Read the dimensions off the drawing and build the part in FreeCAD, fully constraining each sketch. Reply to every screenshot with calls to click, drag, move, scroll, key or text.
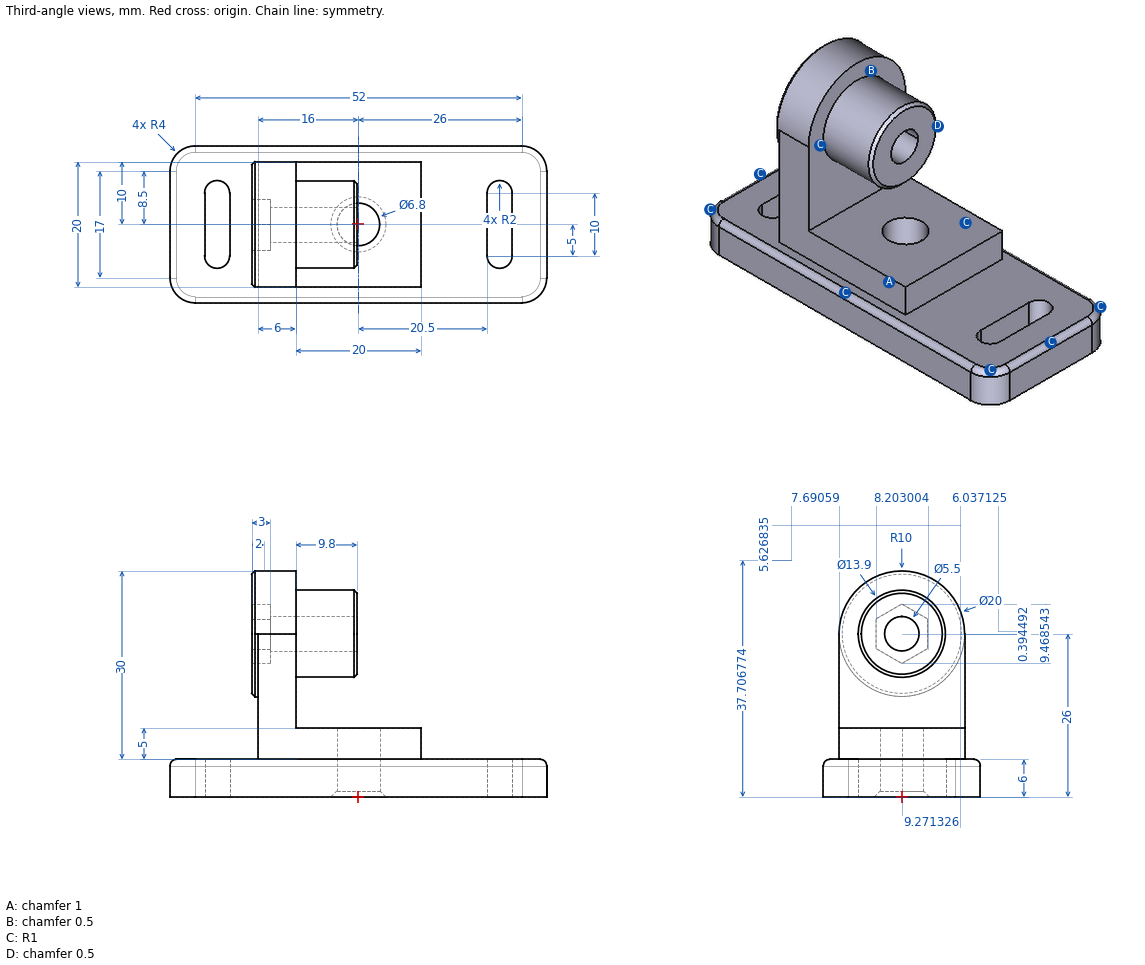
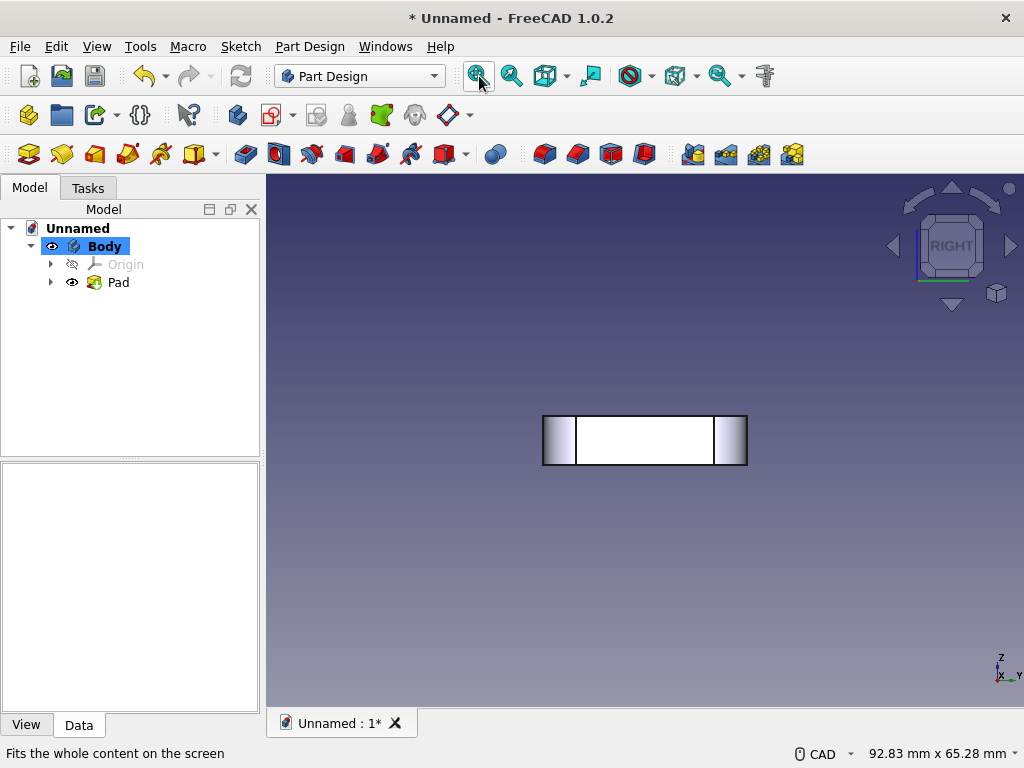
click(623, 456)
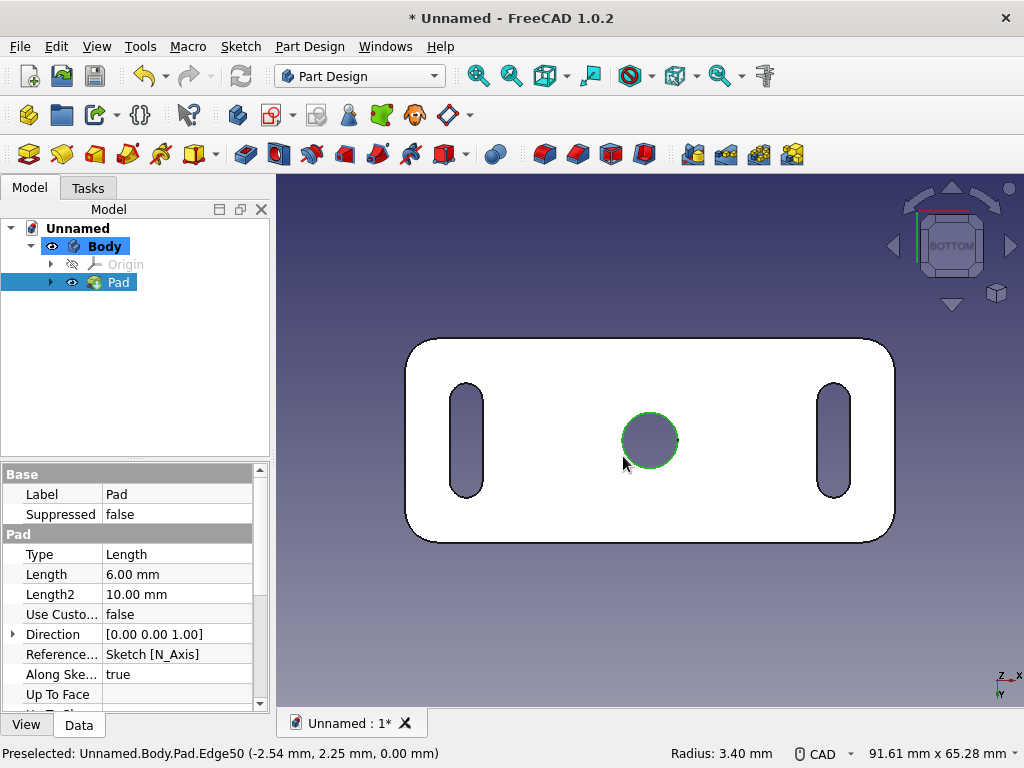
click(578, 154)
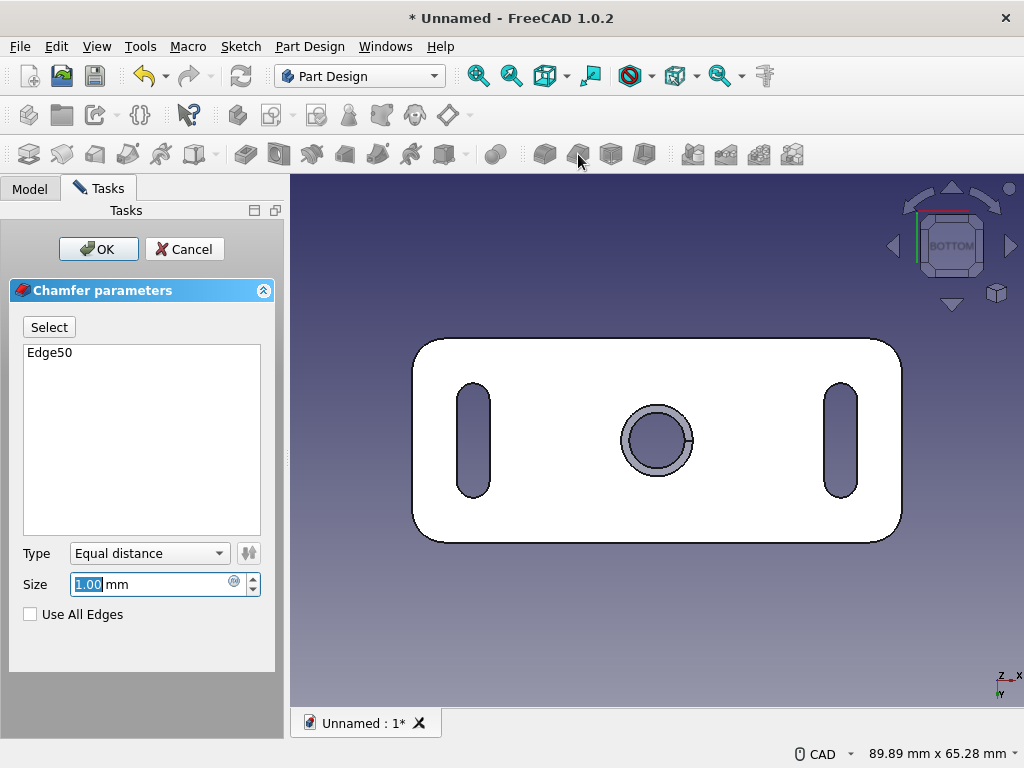
text(1)
key(Tab)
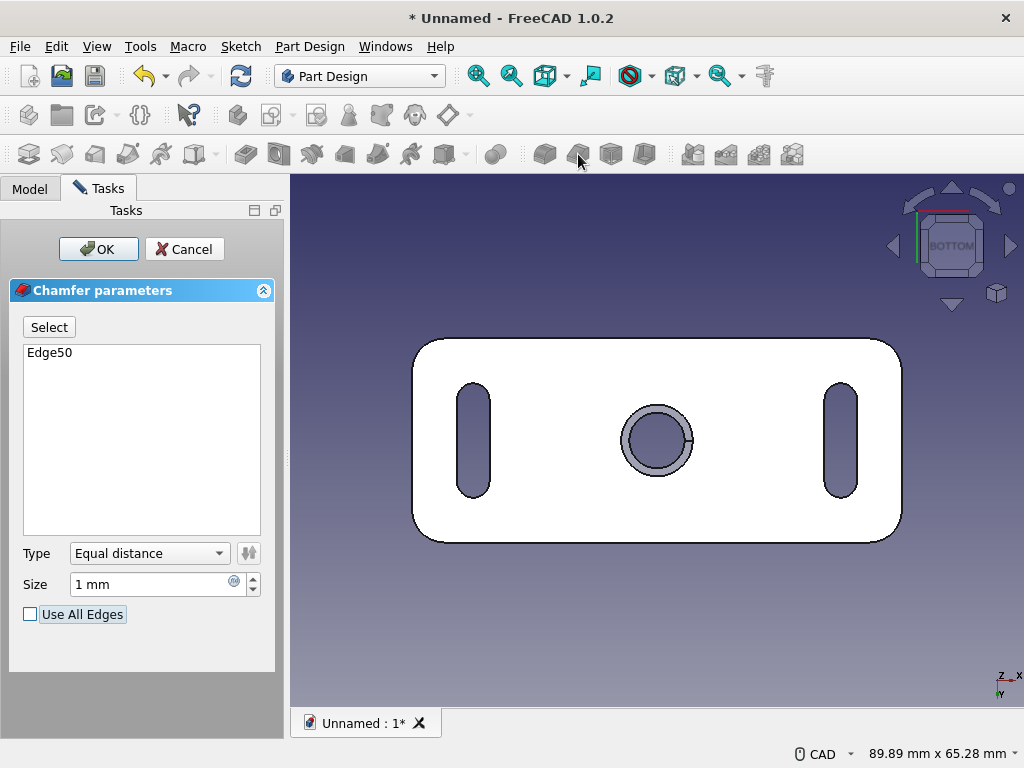
click(99, 249)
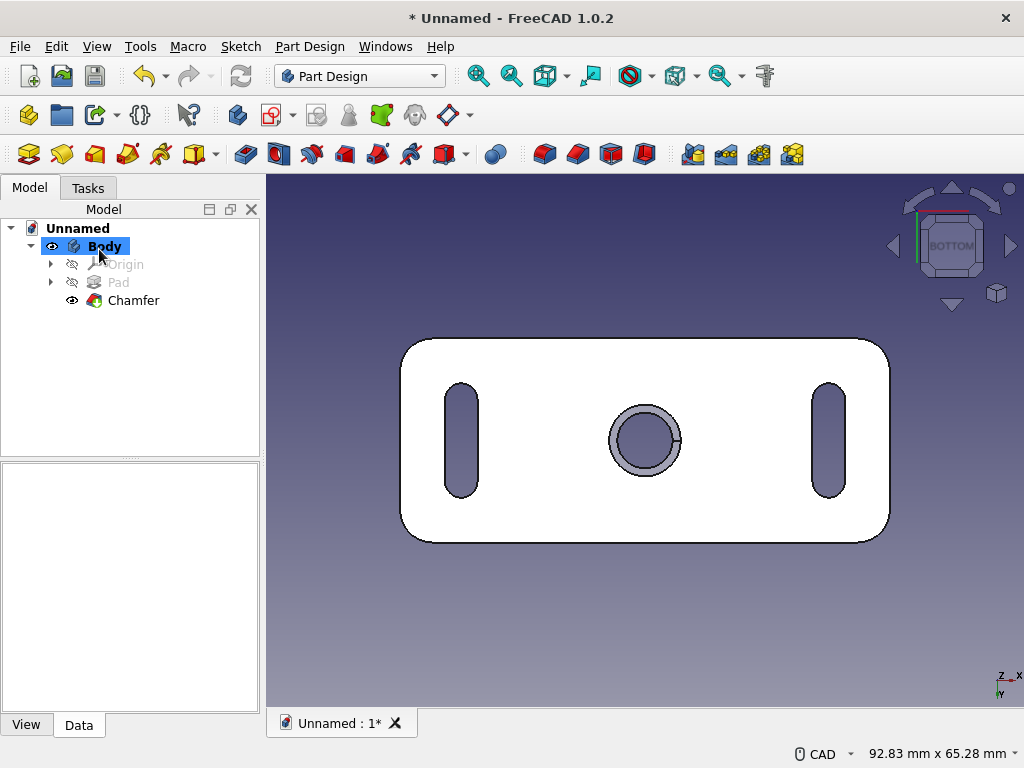
key(0)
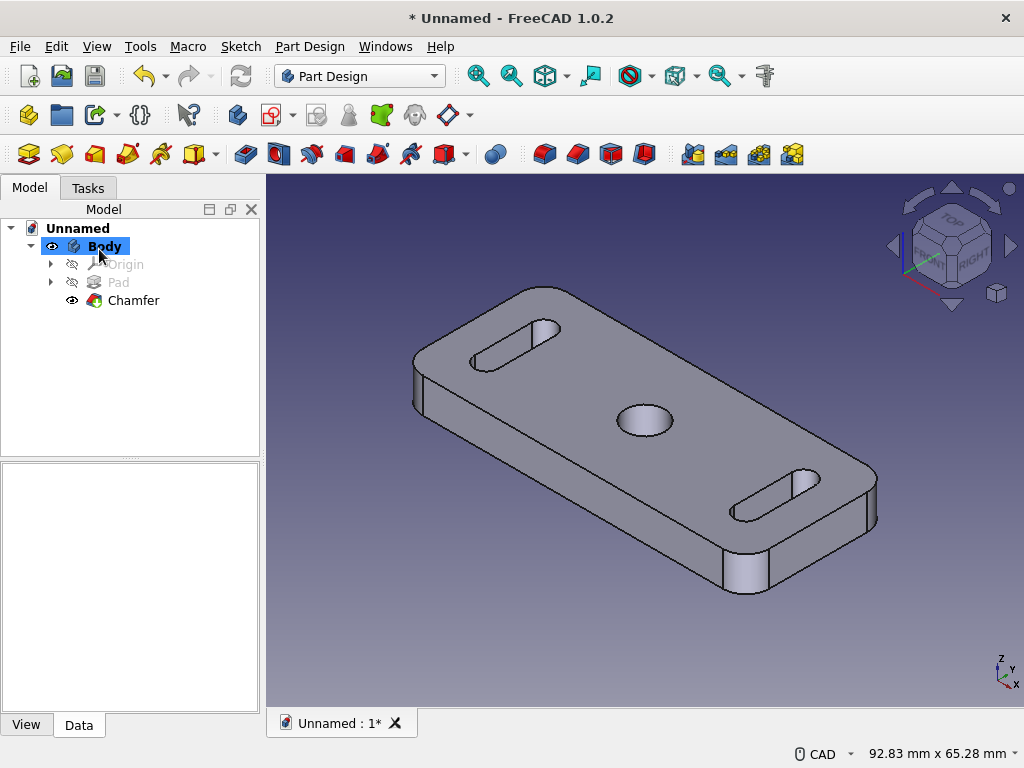
click(616, 379)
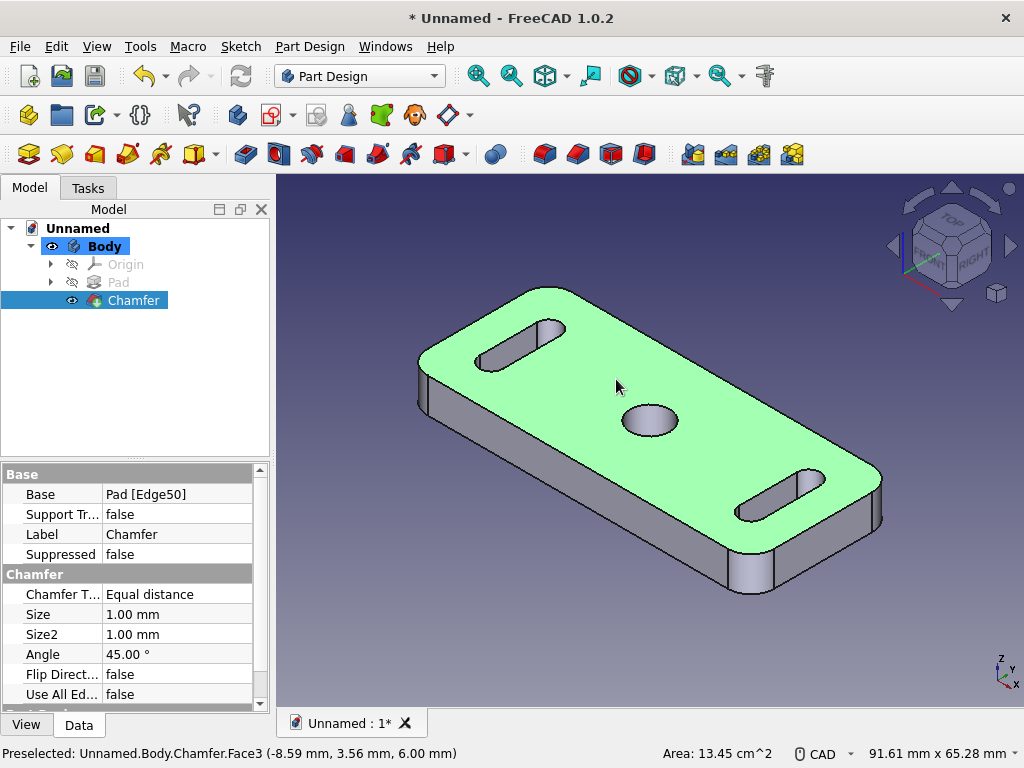
click(270, 116)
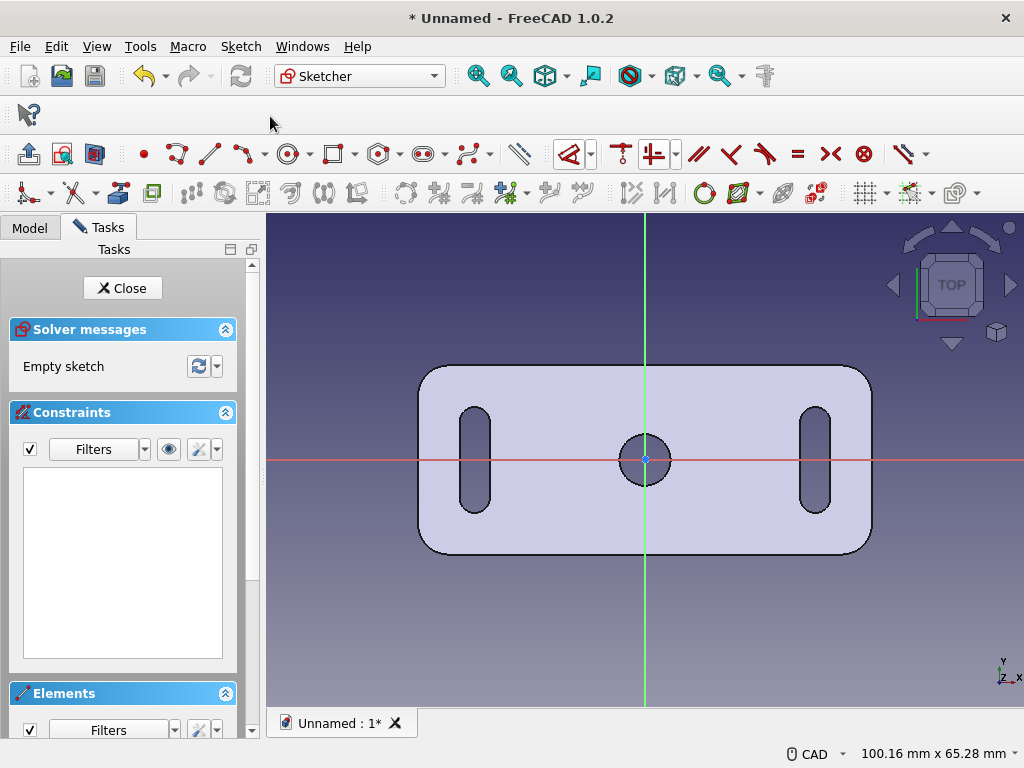
scroll(591, 460, up, 4)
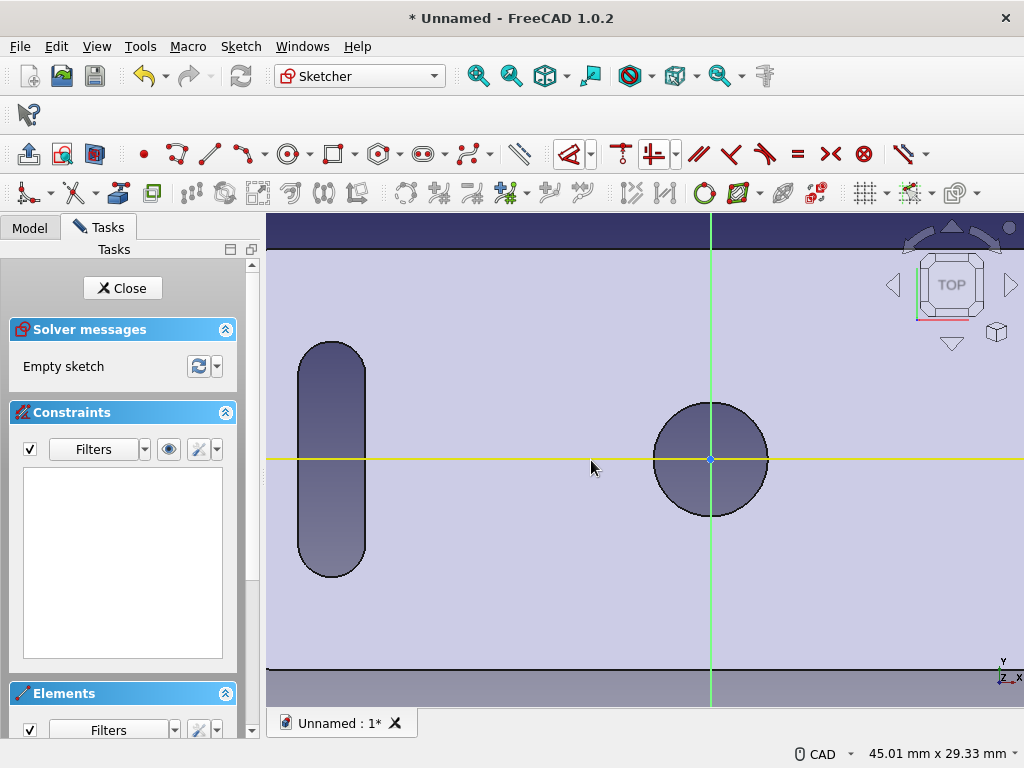
click(332, 154)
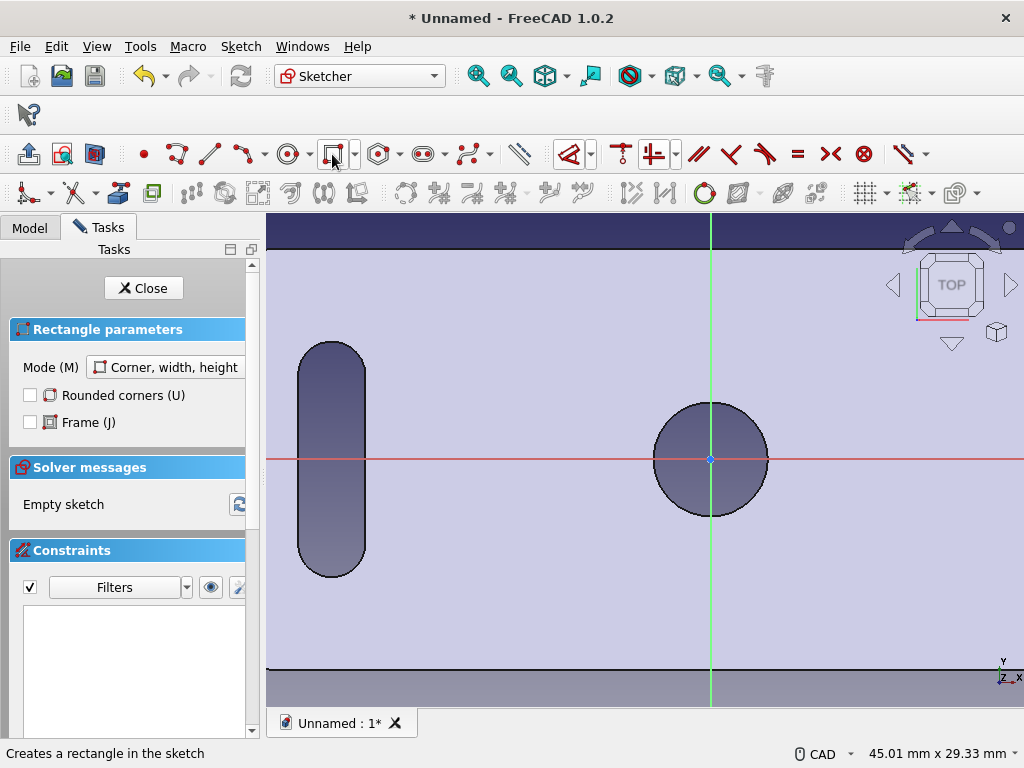
click(441, 291)
move(542, 628)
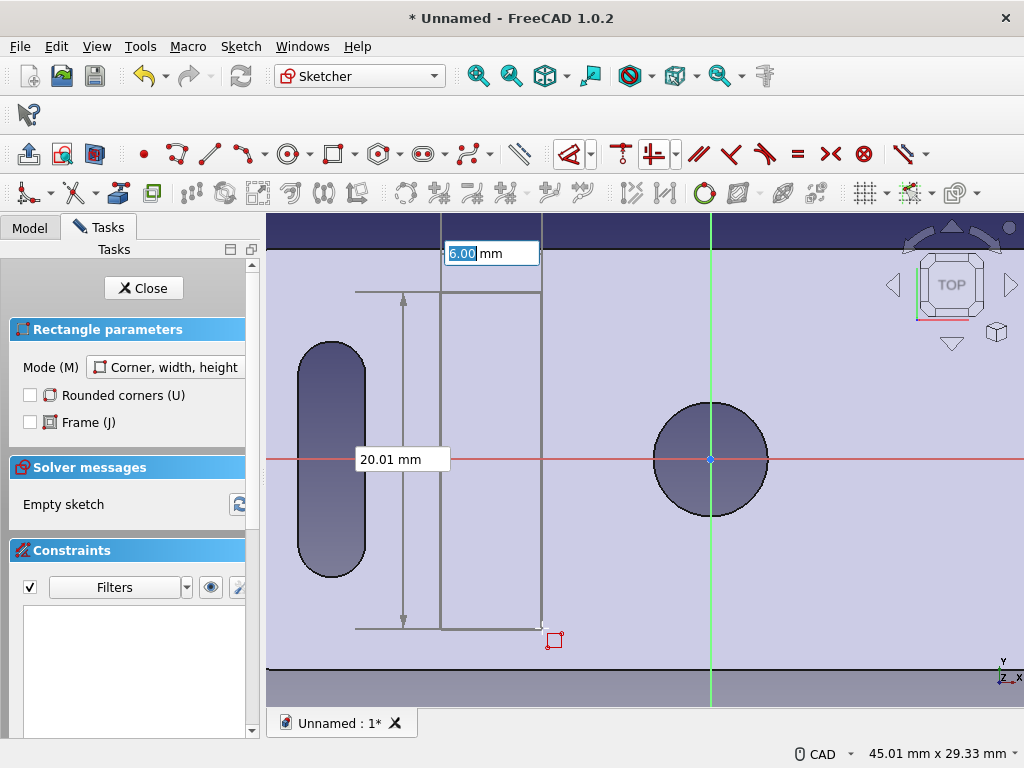
text(6)
key(Tab)
text(20)
key(Return)
key(Escape)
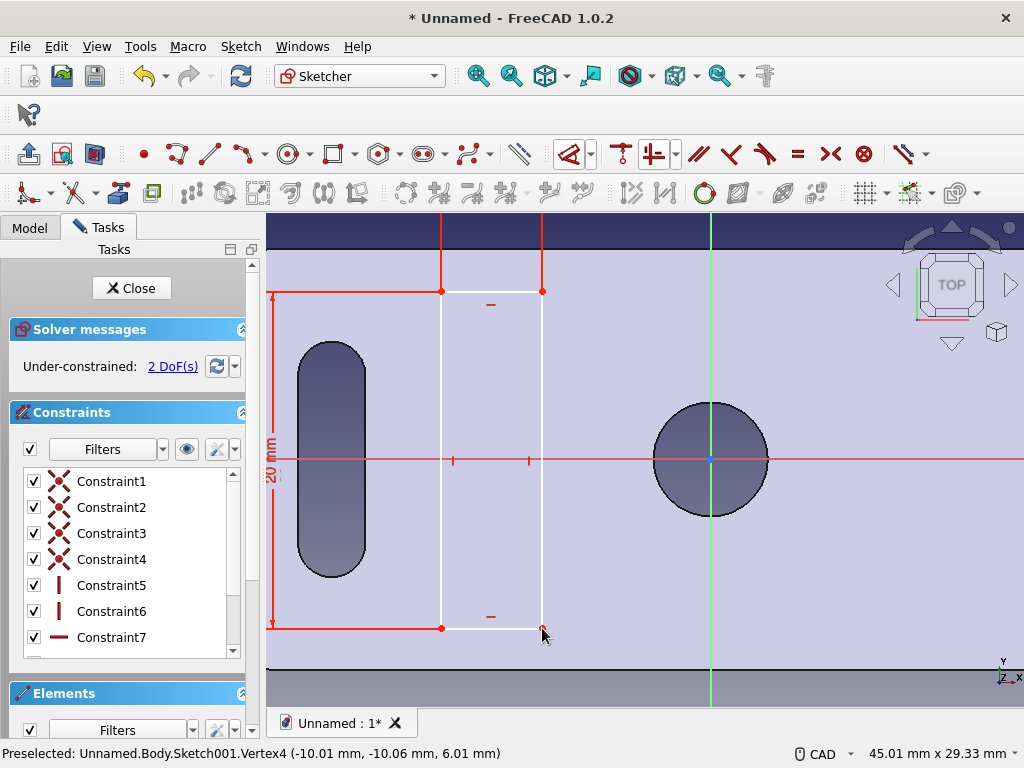
click(441, 292)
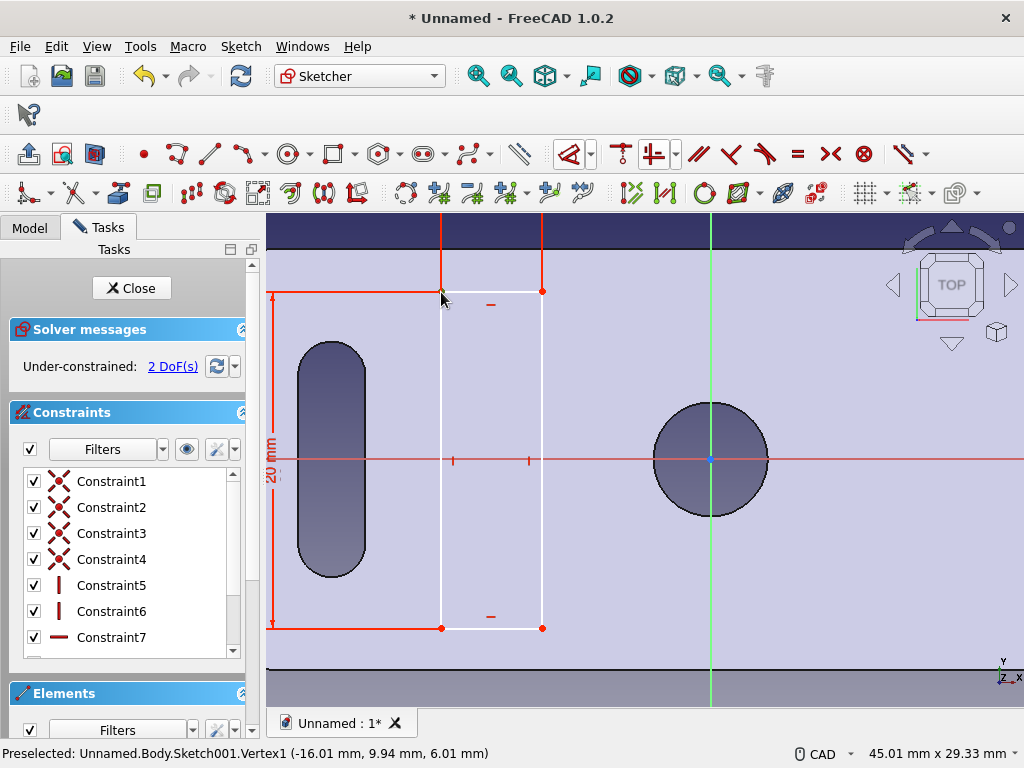
click(590, 154)